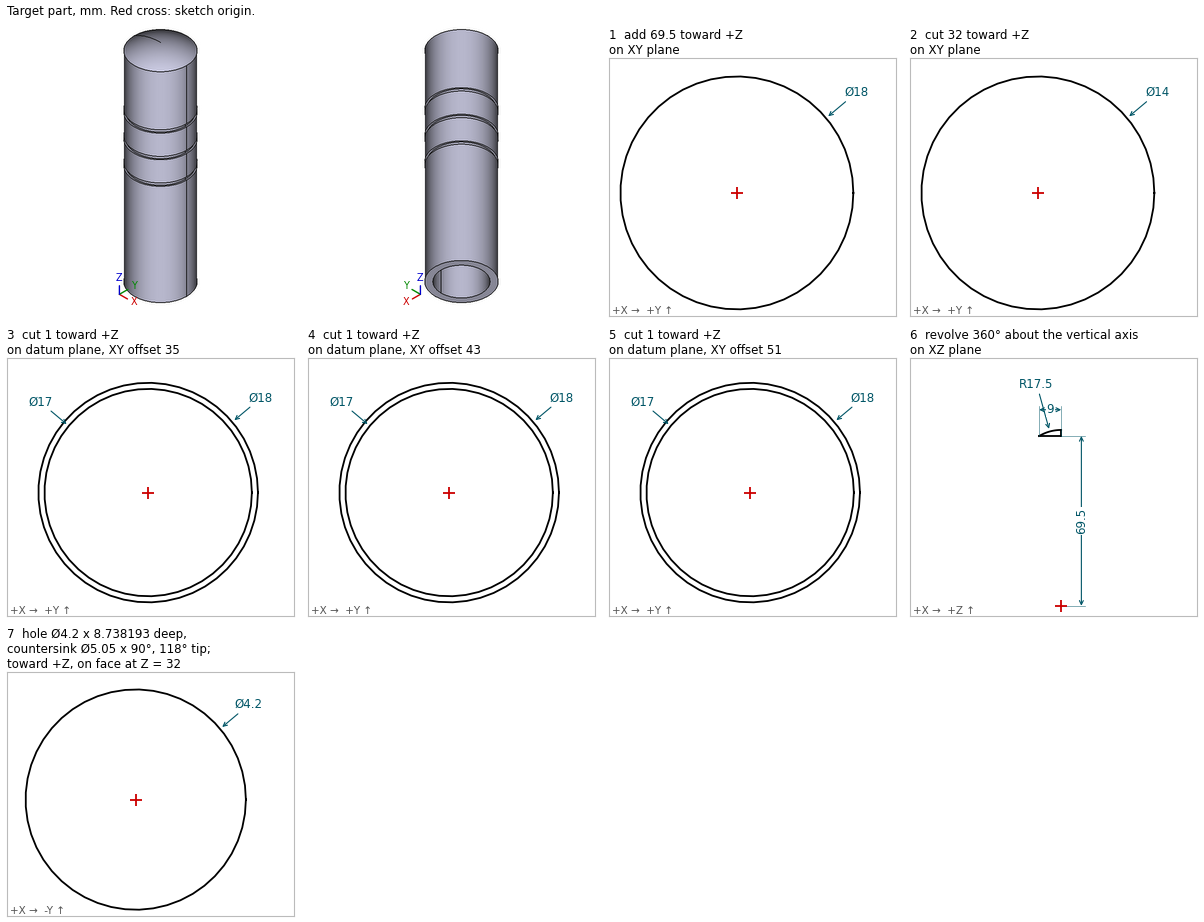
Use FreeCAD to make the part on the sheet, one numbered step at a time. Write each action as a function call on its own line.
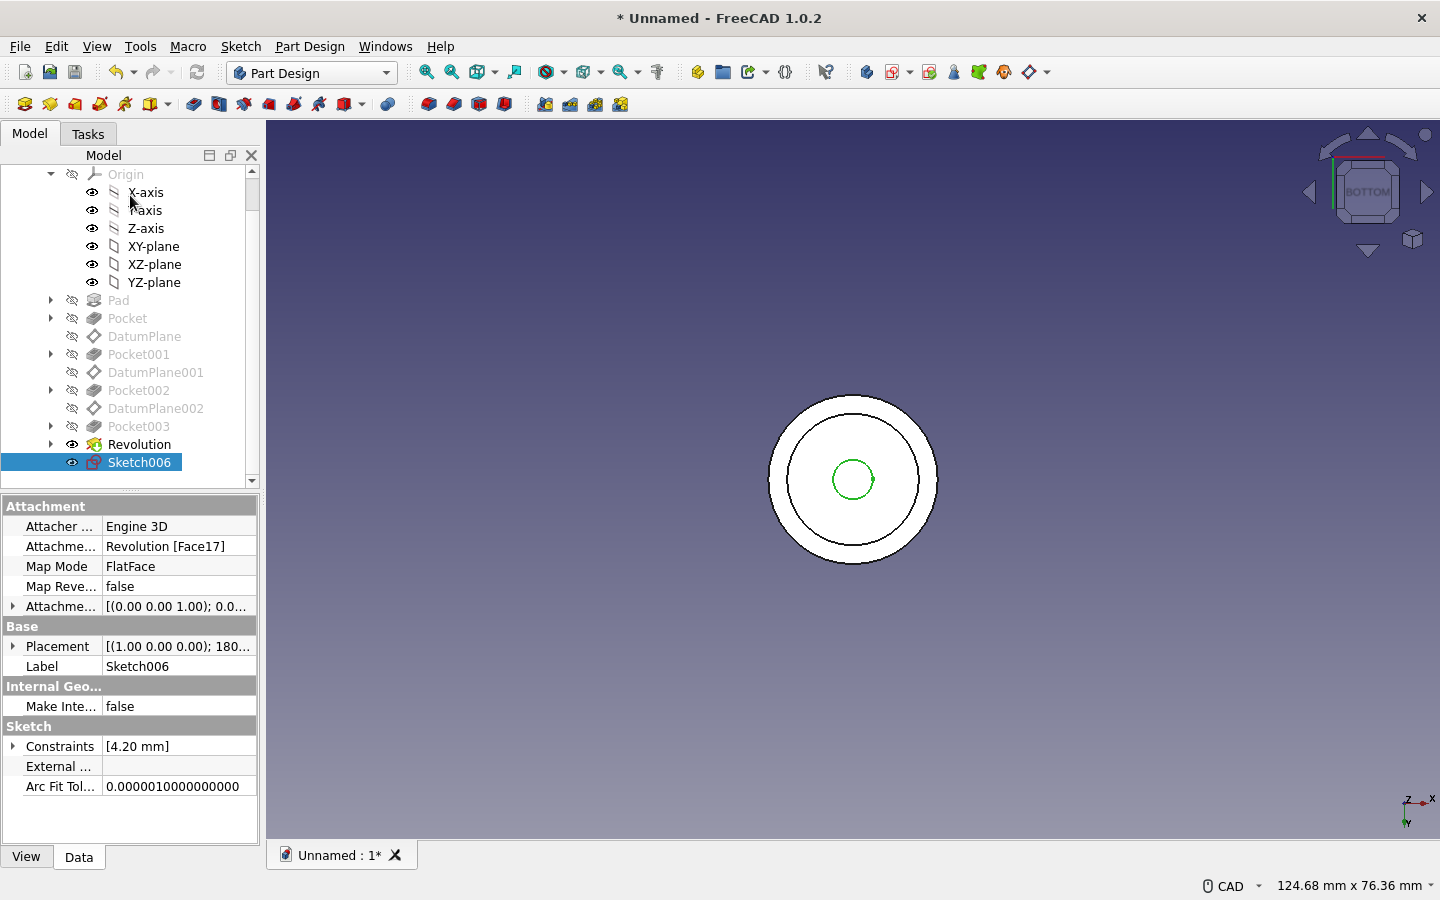
click(219, 104)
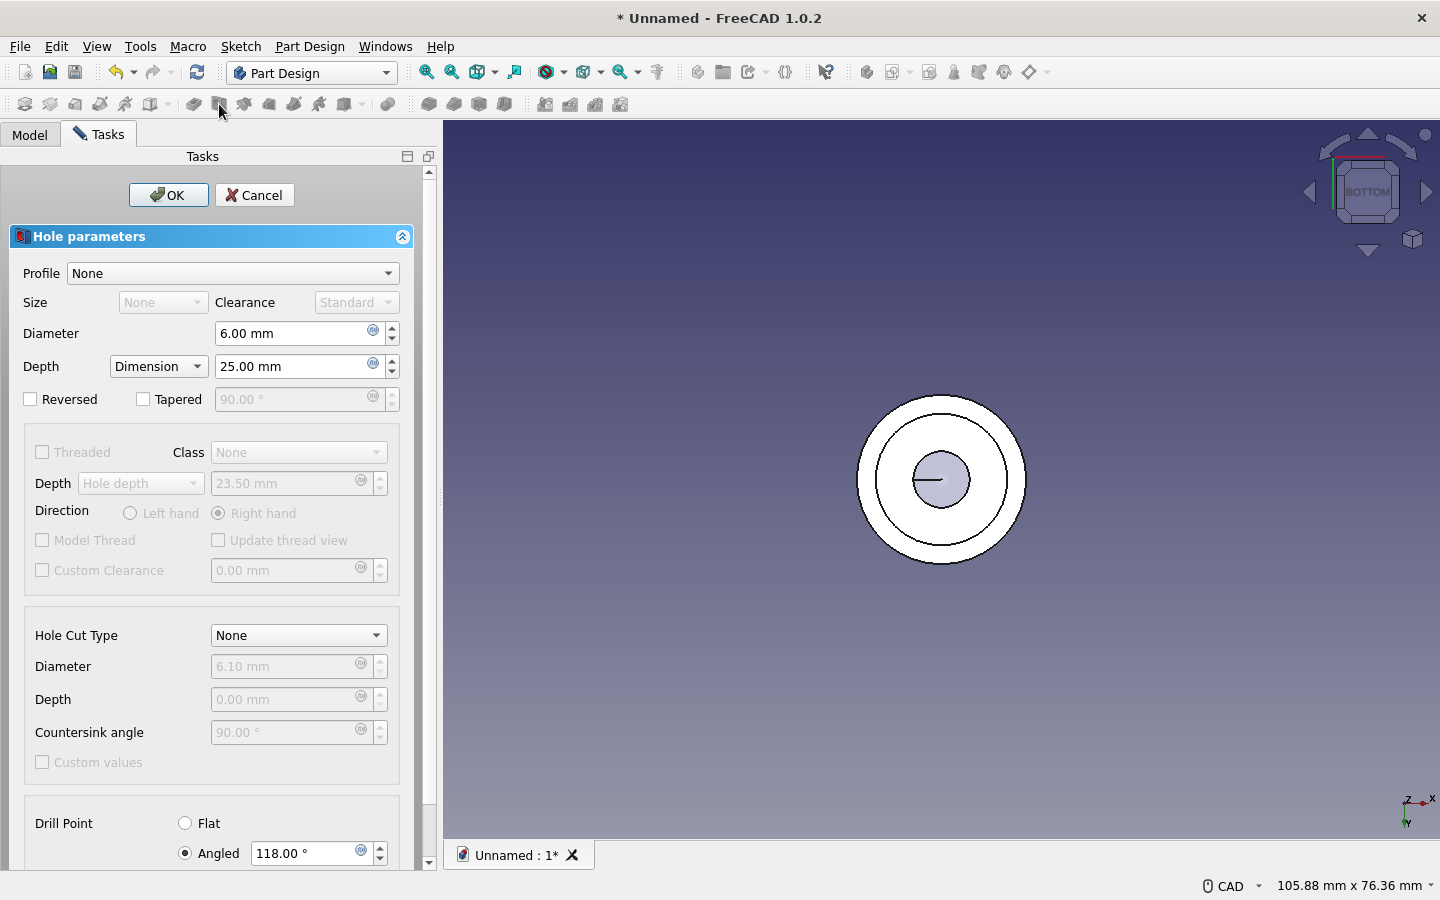
triple_click(300, 334)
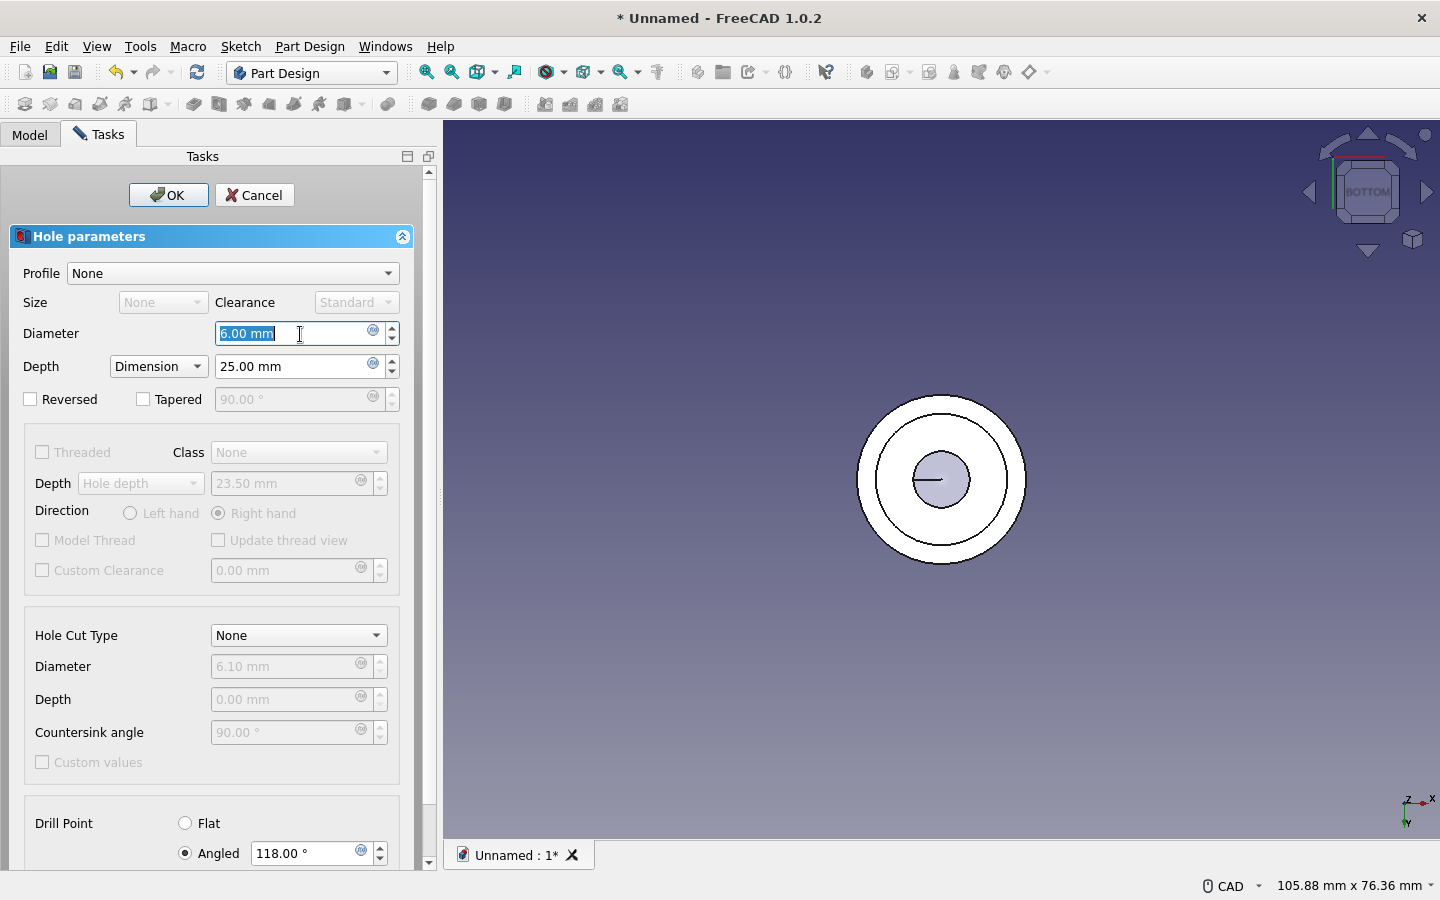
text(4.2)
key(Tab)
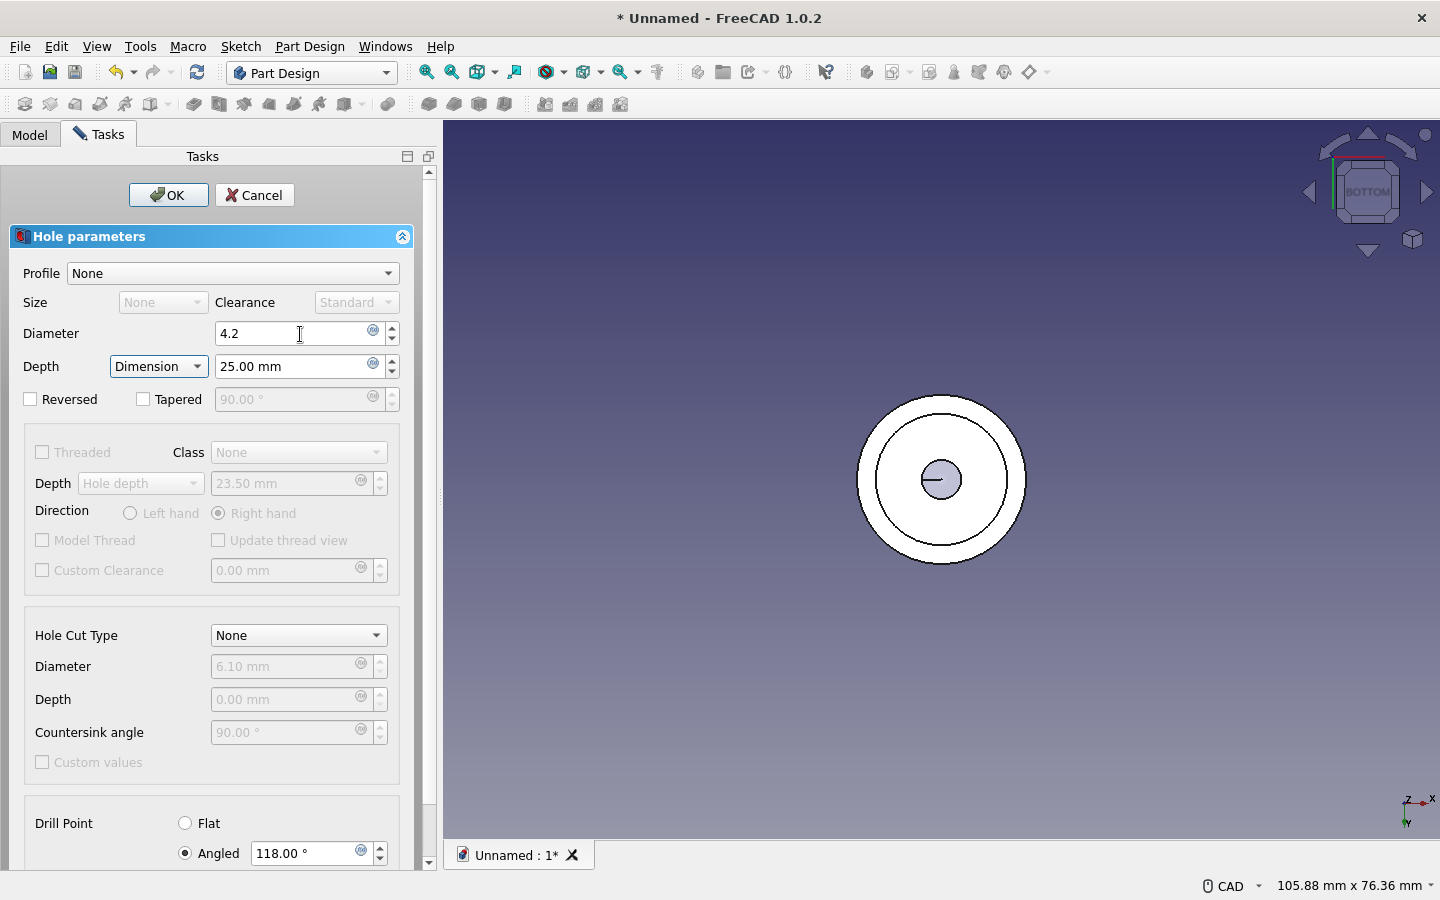
triple_click(300, 366)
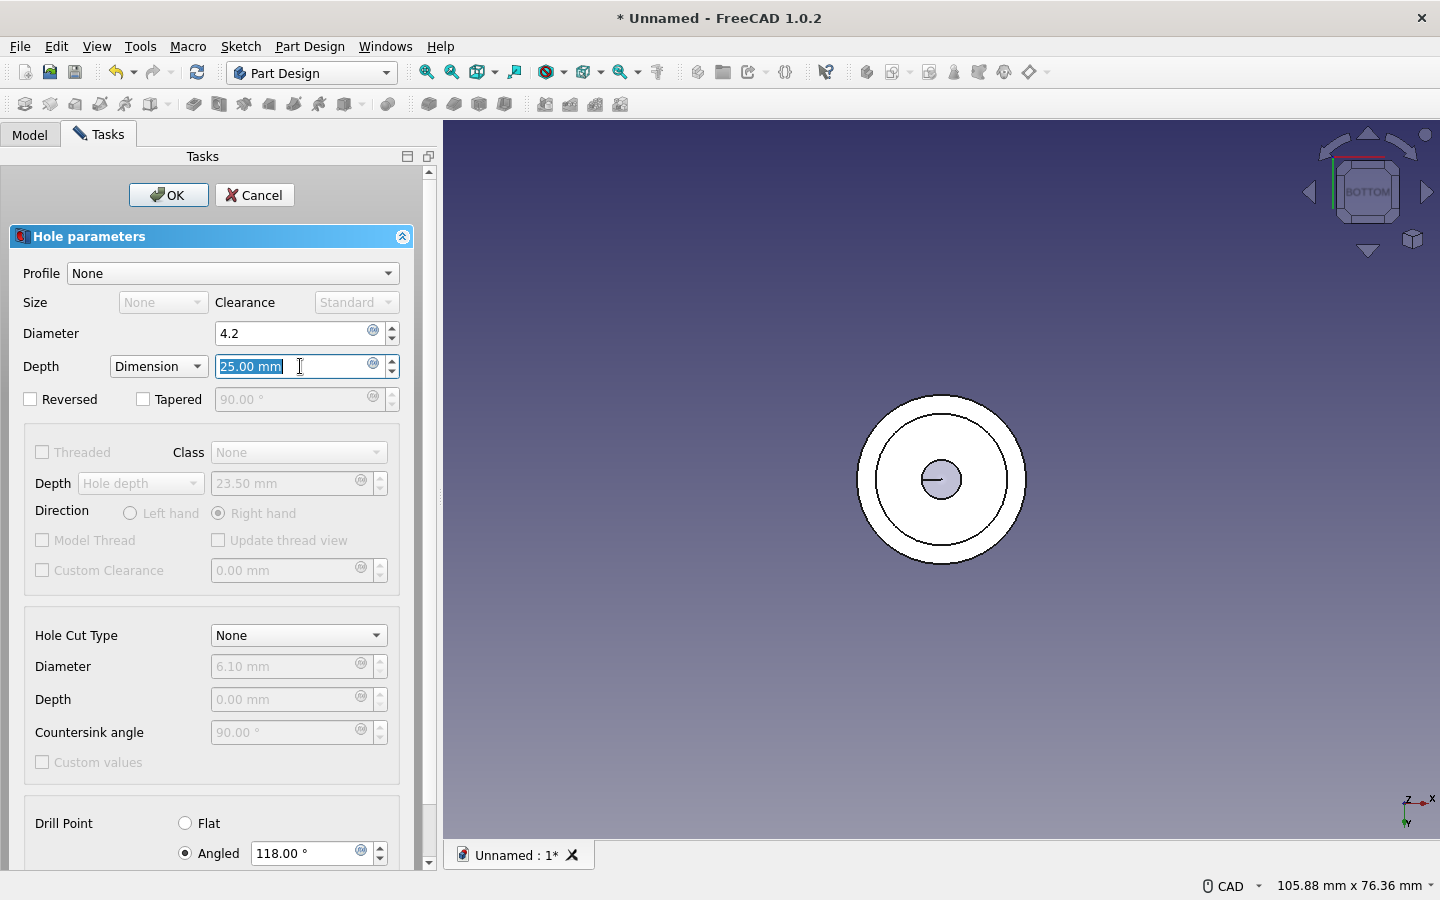
text(8.738193)
key(Tab)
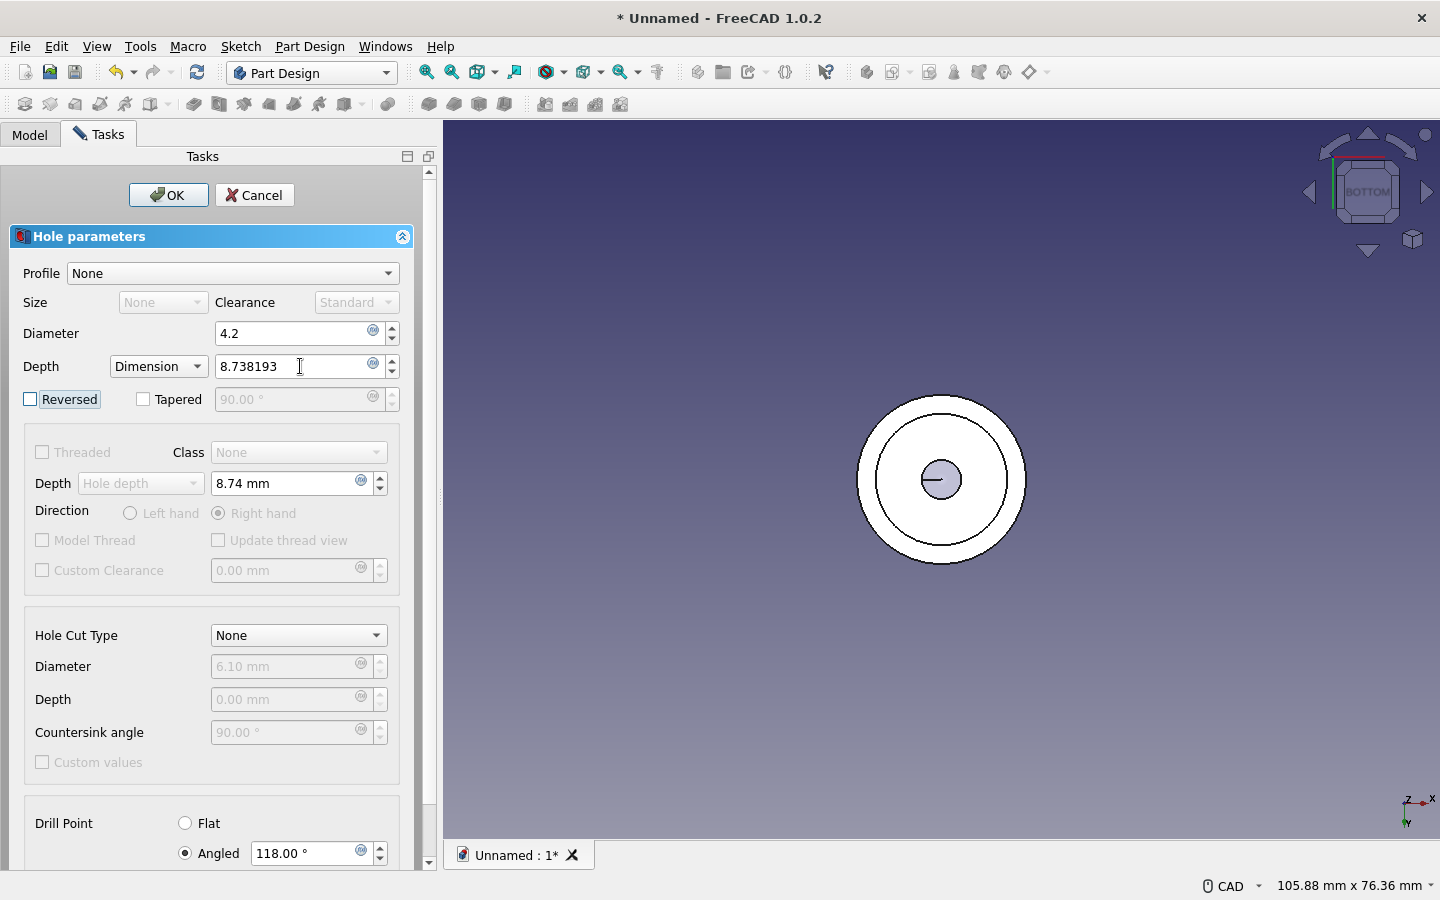
click(300, 636)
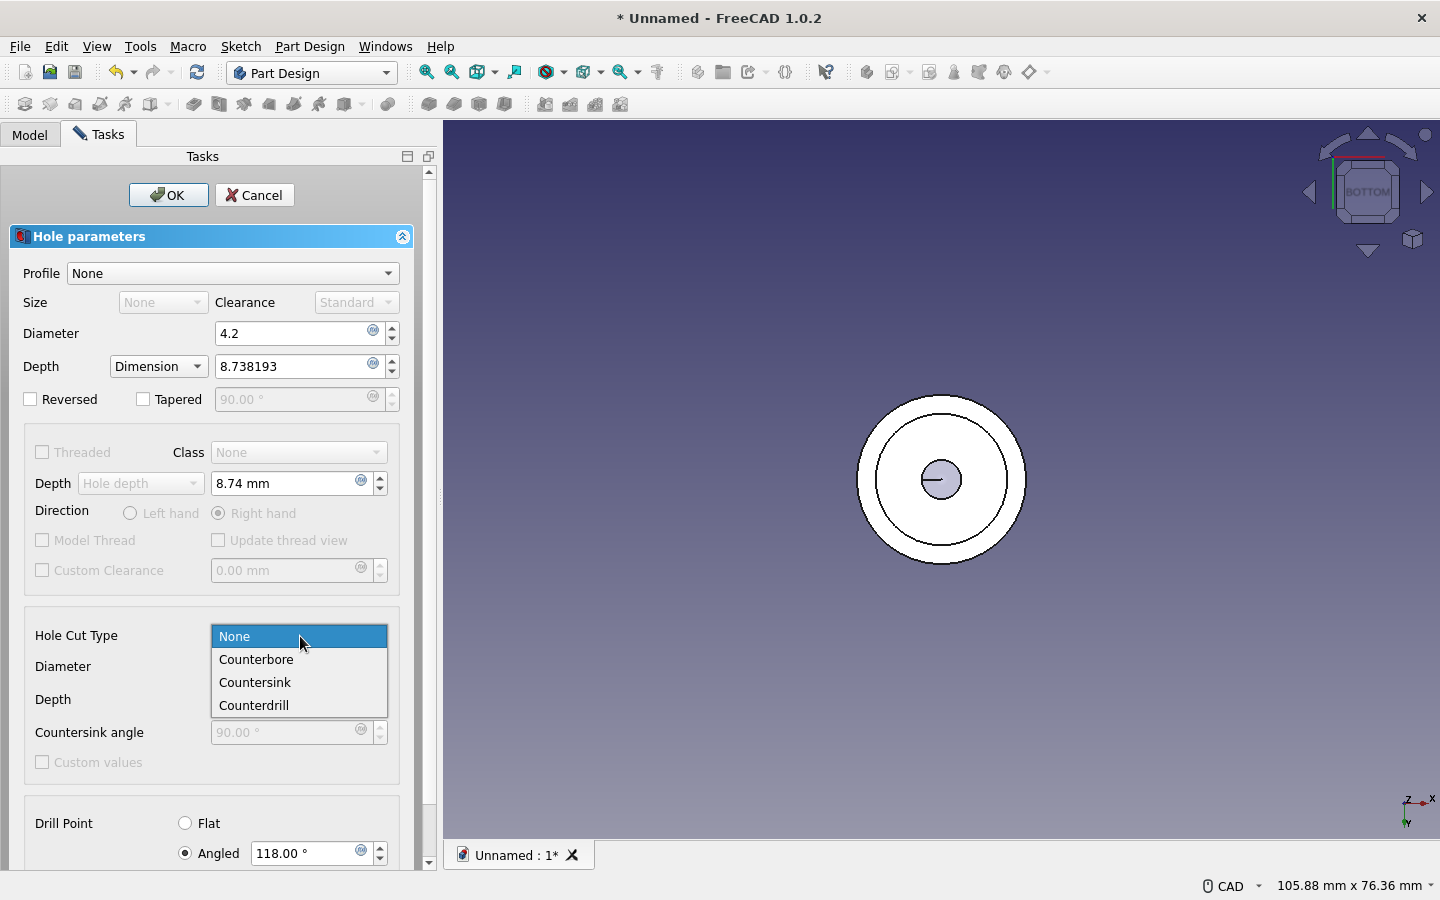
click(298, 682)